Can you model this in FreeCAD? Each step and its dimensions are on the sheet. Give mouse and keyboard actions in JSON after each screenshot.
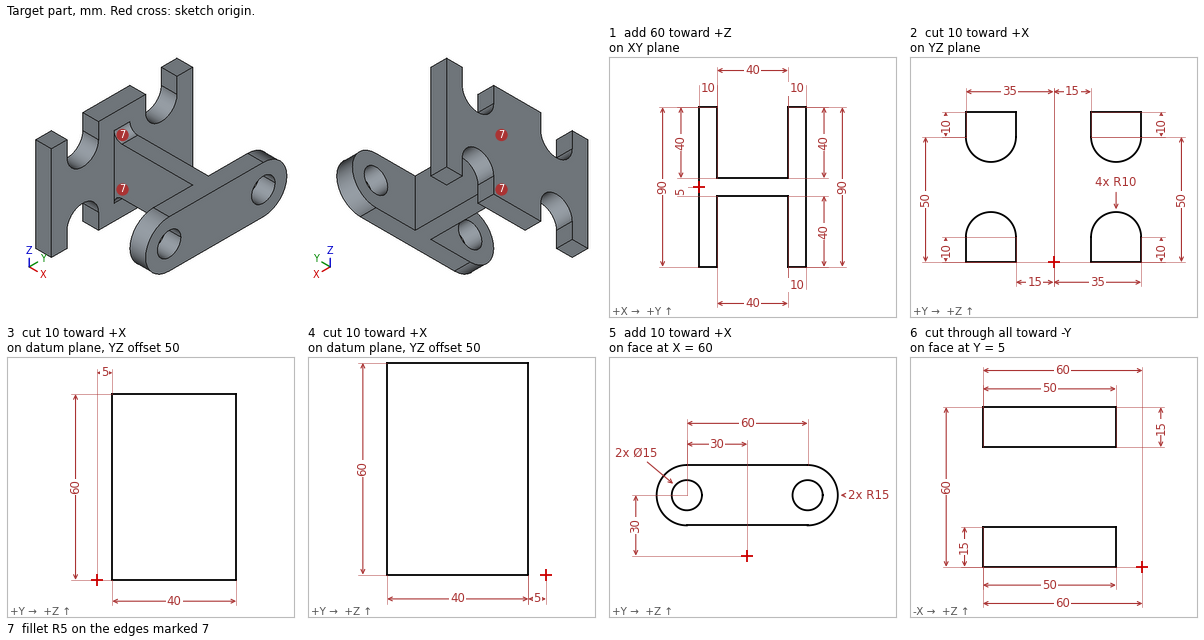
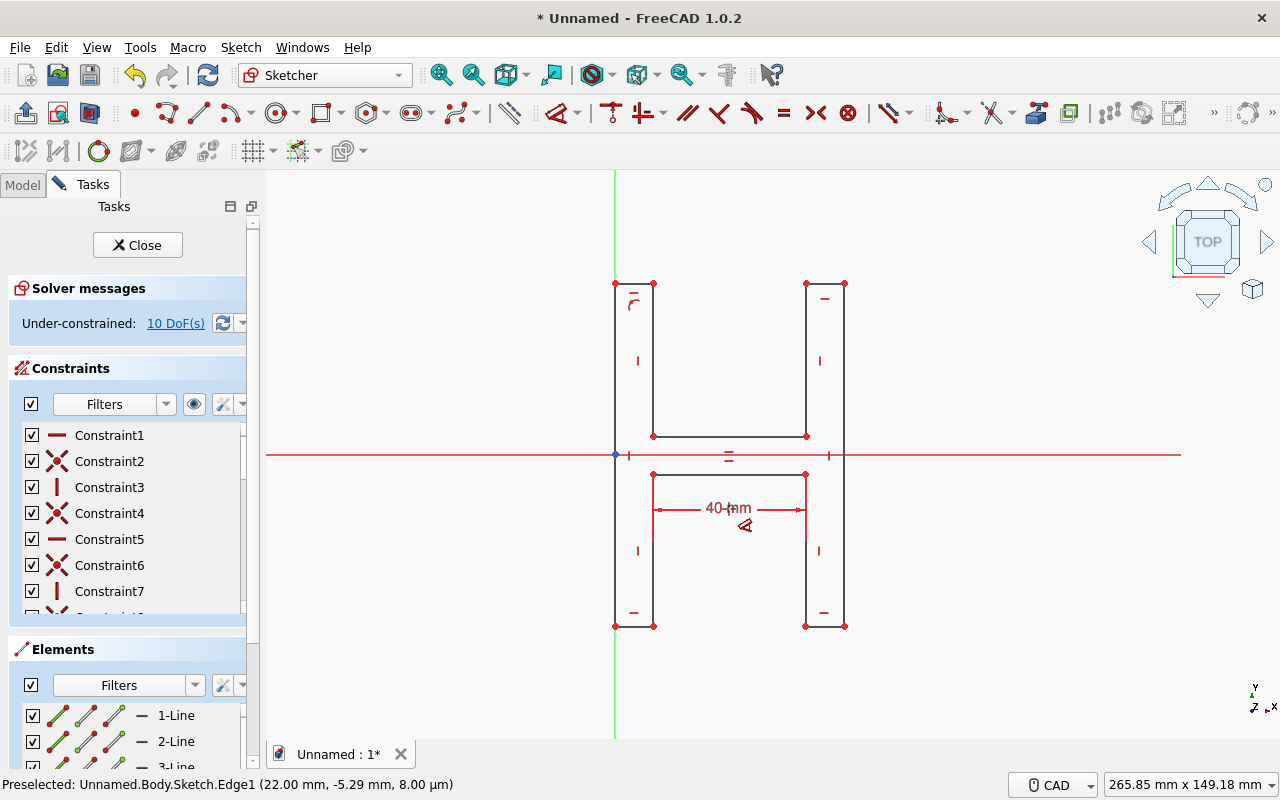
{"action": "left_click", "coordinate": [806, 521]}
{"action": "left_click", "coordinate": [772, 551]}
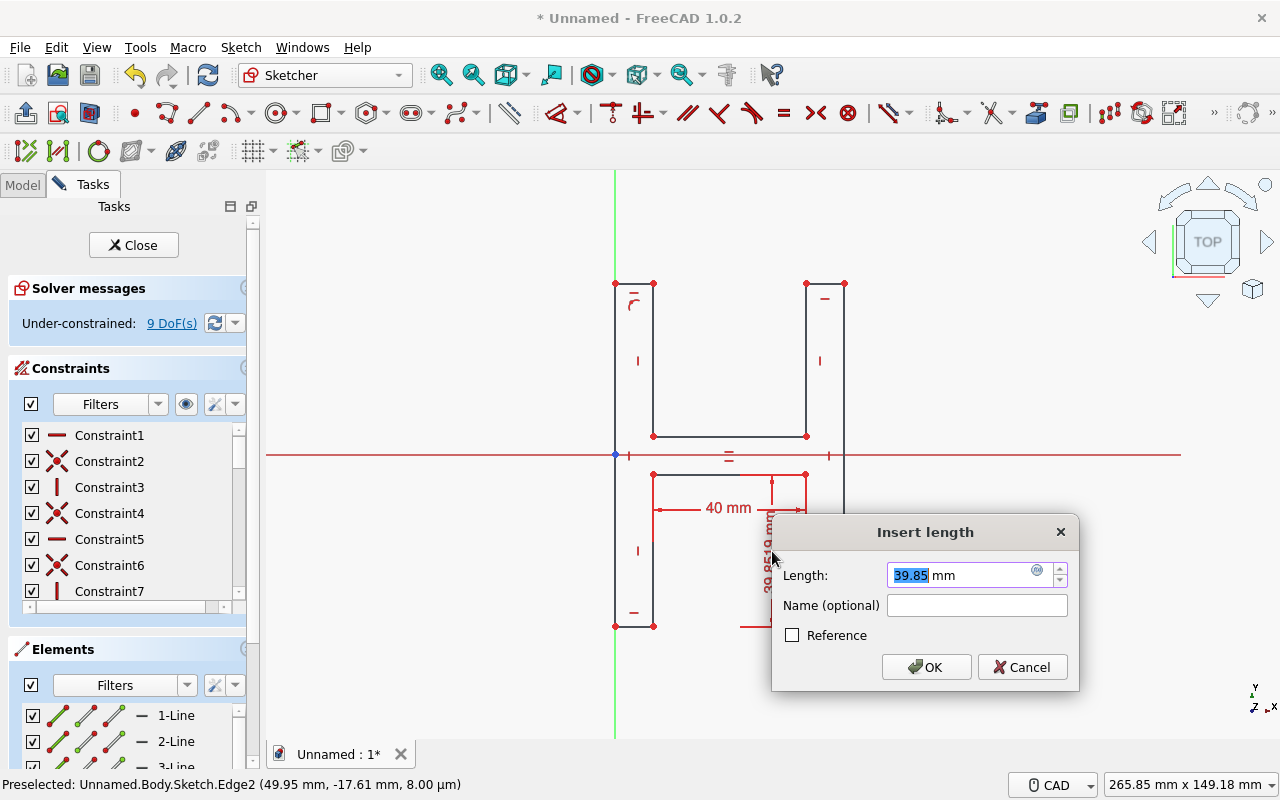
{"action": "type", "text": "40"}
{"action": "key", "text": "Return"}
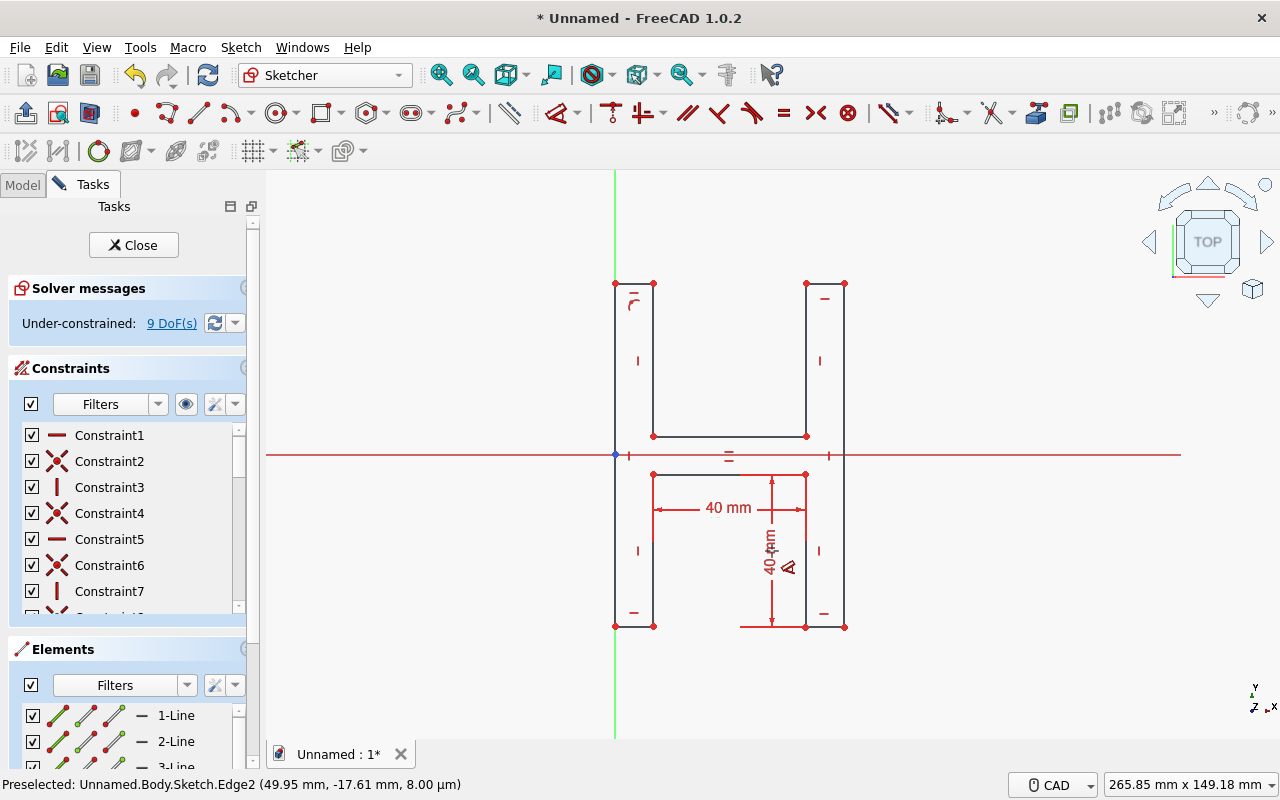
{"action": "left_click", "coordinate": [817, 627]}
{"action": "left_click", "coordinate": [825, 661]}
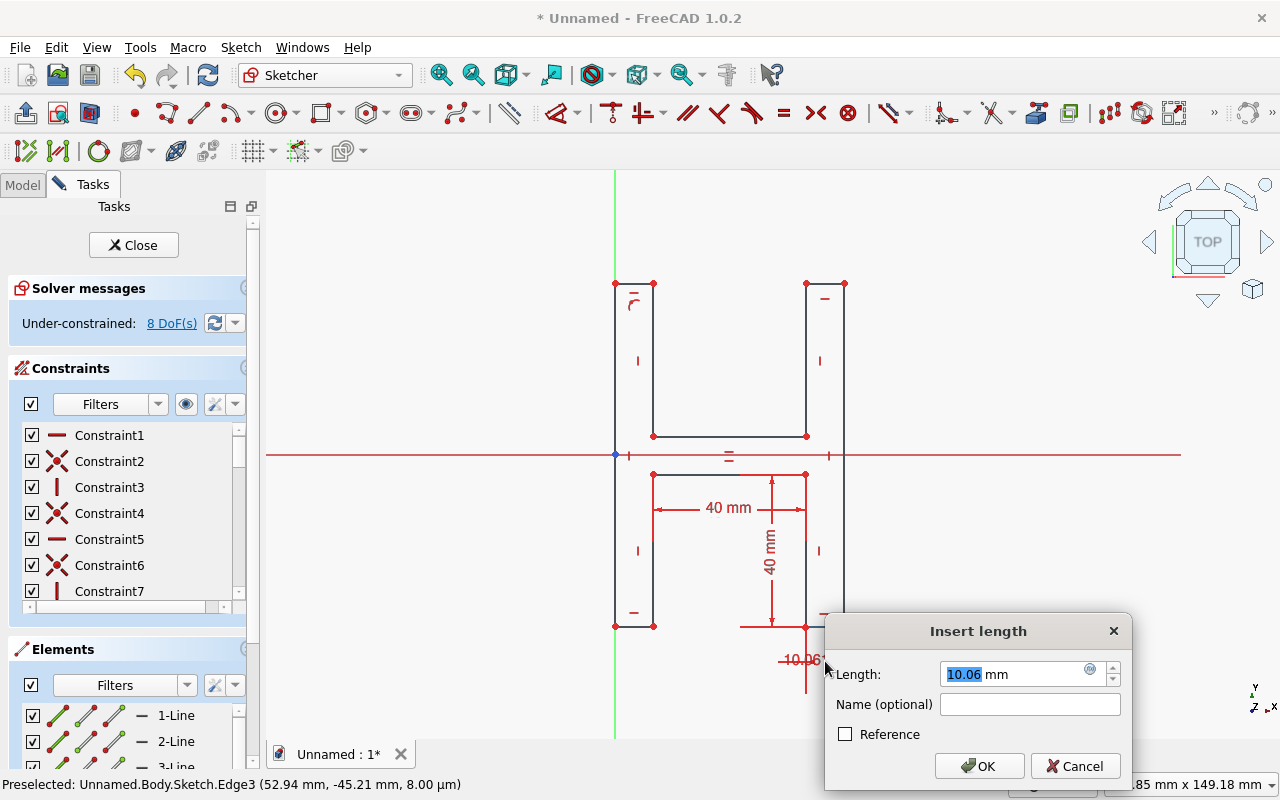
{"action": "type", "text": "10"}
{"action": "key", "text": "Return"}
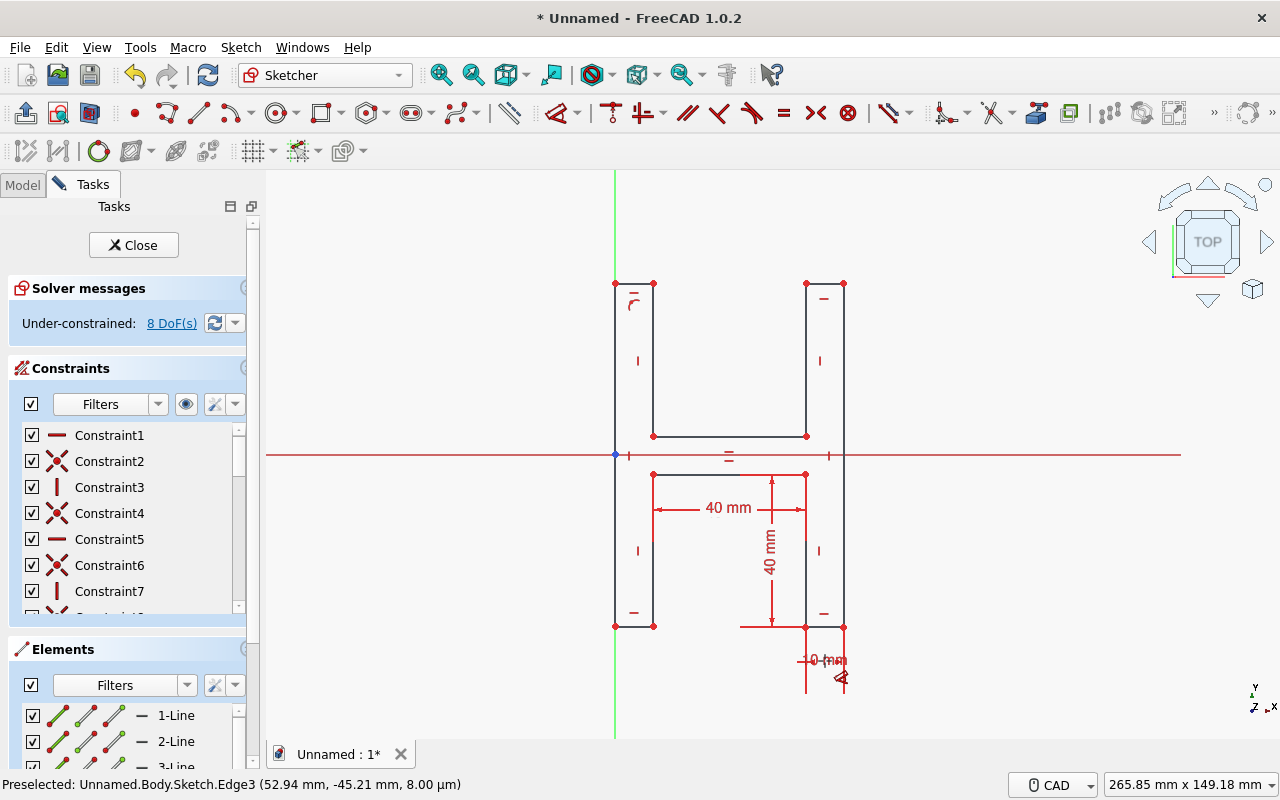
{"action": "left_click", "coordinate": [844, 524]}
{"action": "left_click", "coordinate": [878, 377]}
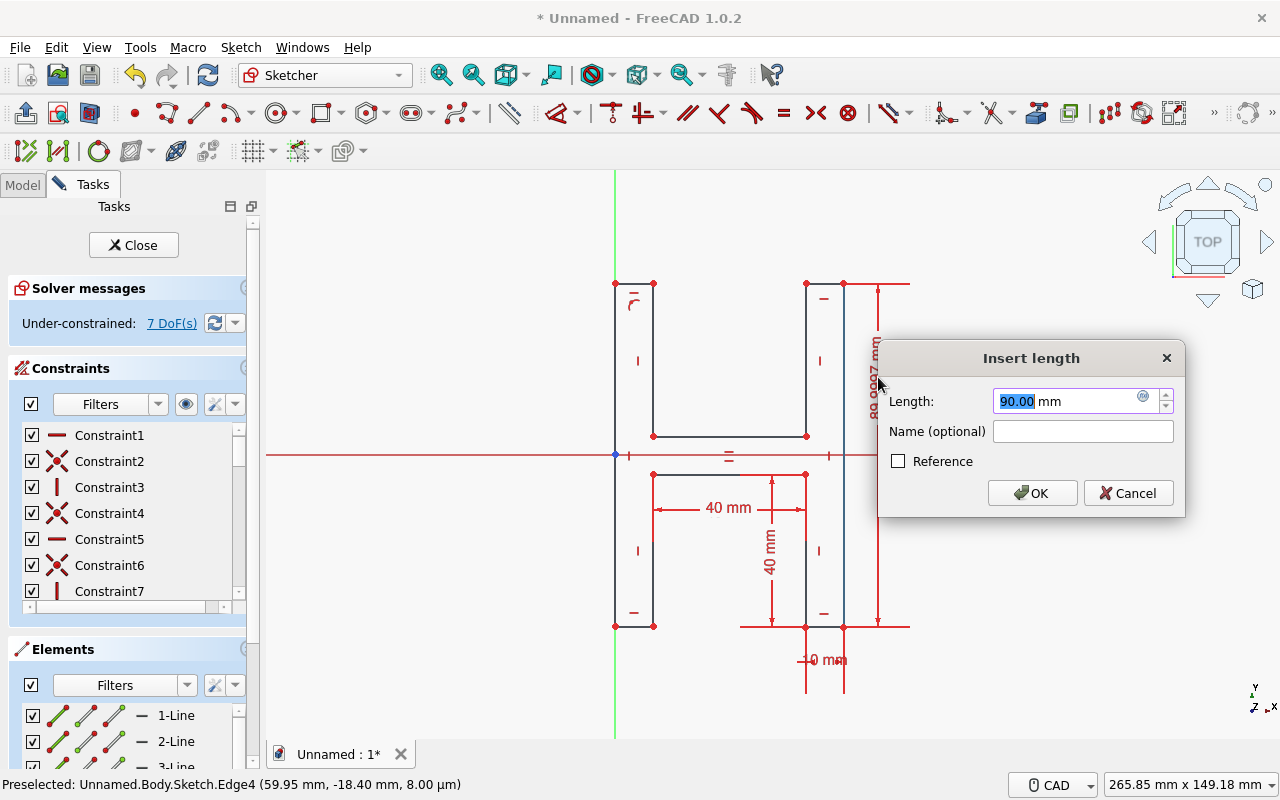
{"action": "type", "text": "90"}
{"action": "key", "text": "Return"}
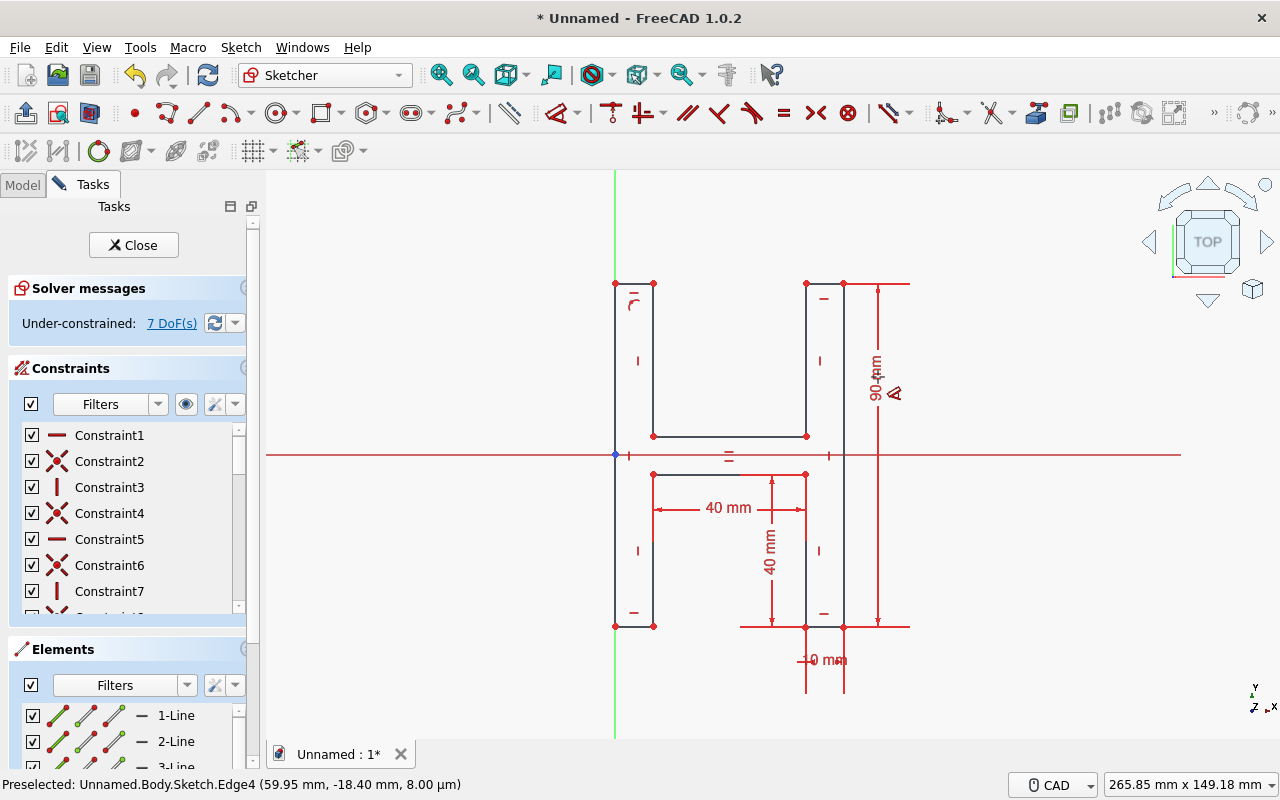
{"action": "left_click", "coordinate": [832, 284]}
{"action": "left_click", "coordinate": [825, 250]}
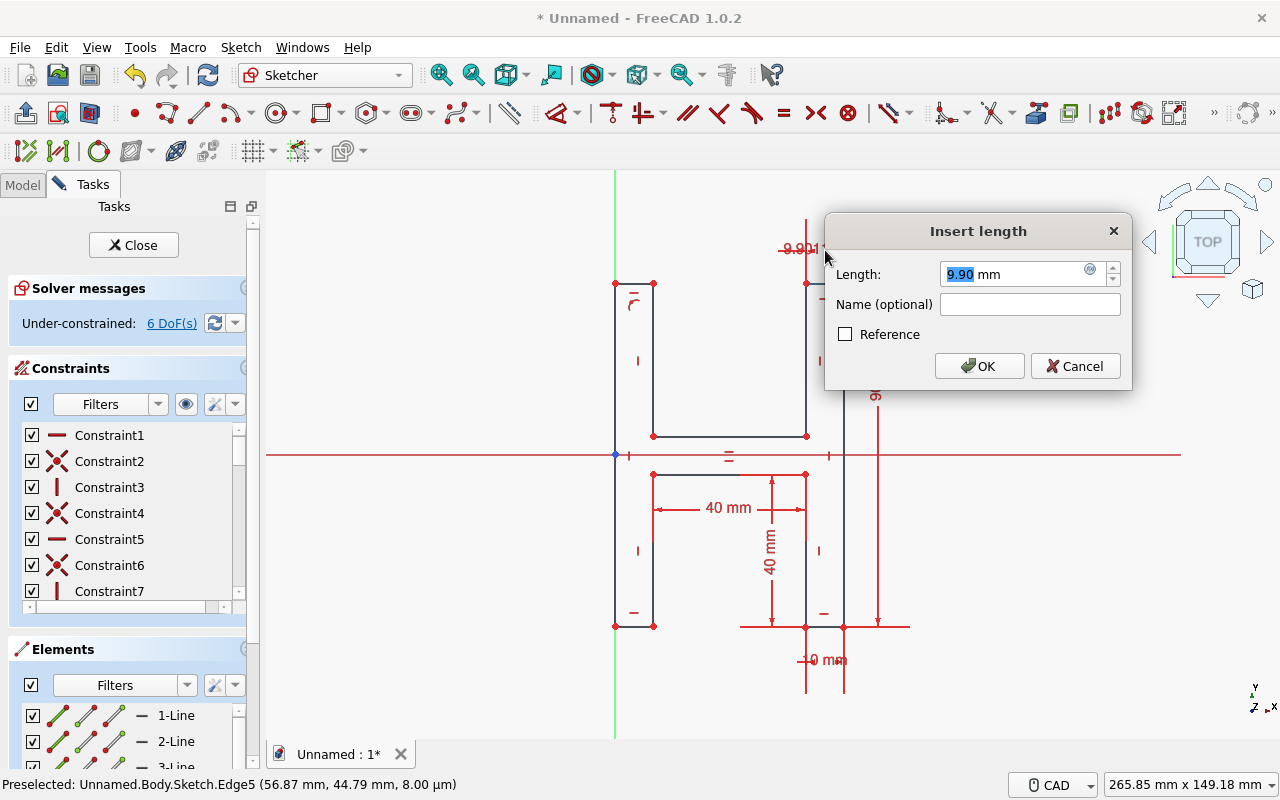
{"action": "type", "text": "10"}
{"action": "key", "text": "Return"}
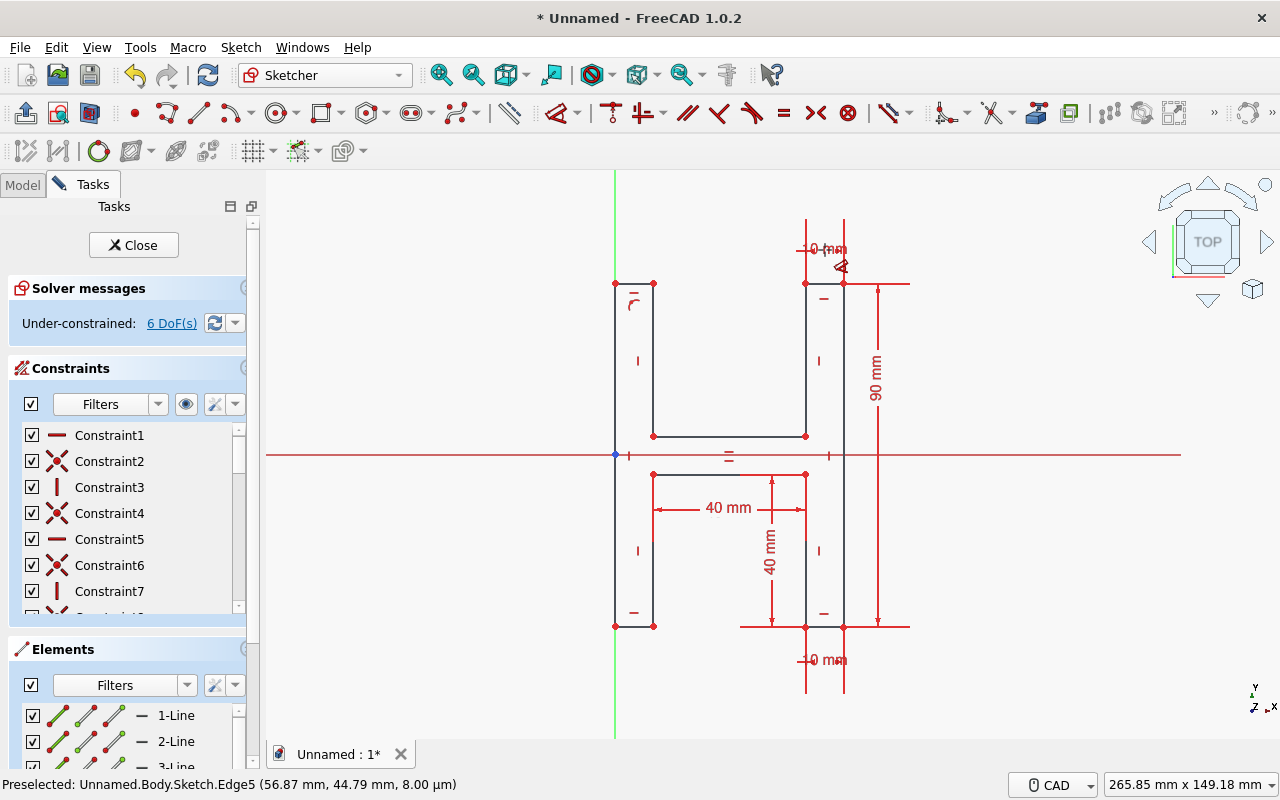
{"action": "left_click", "coordinate": [806, 330]}
{"action": "left_click", "coordinate": [772, 360]}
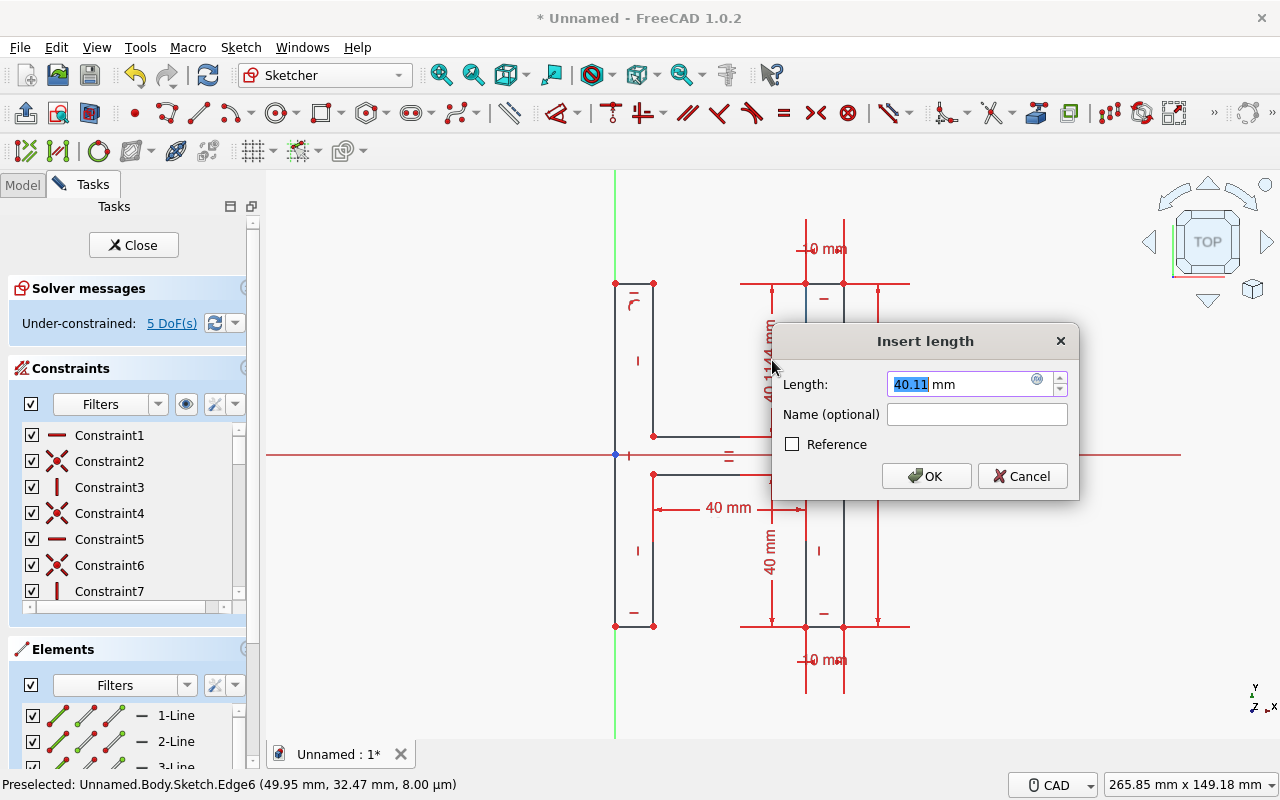
{"action": "type", "text": "40"}
{"action": "key", "text": "Return"}